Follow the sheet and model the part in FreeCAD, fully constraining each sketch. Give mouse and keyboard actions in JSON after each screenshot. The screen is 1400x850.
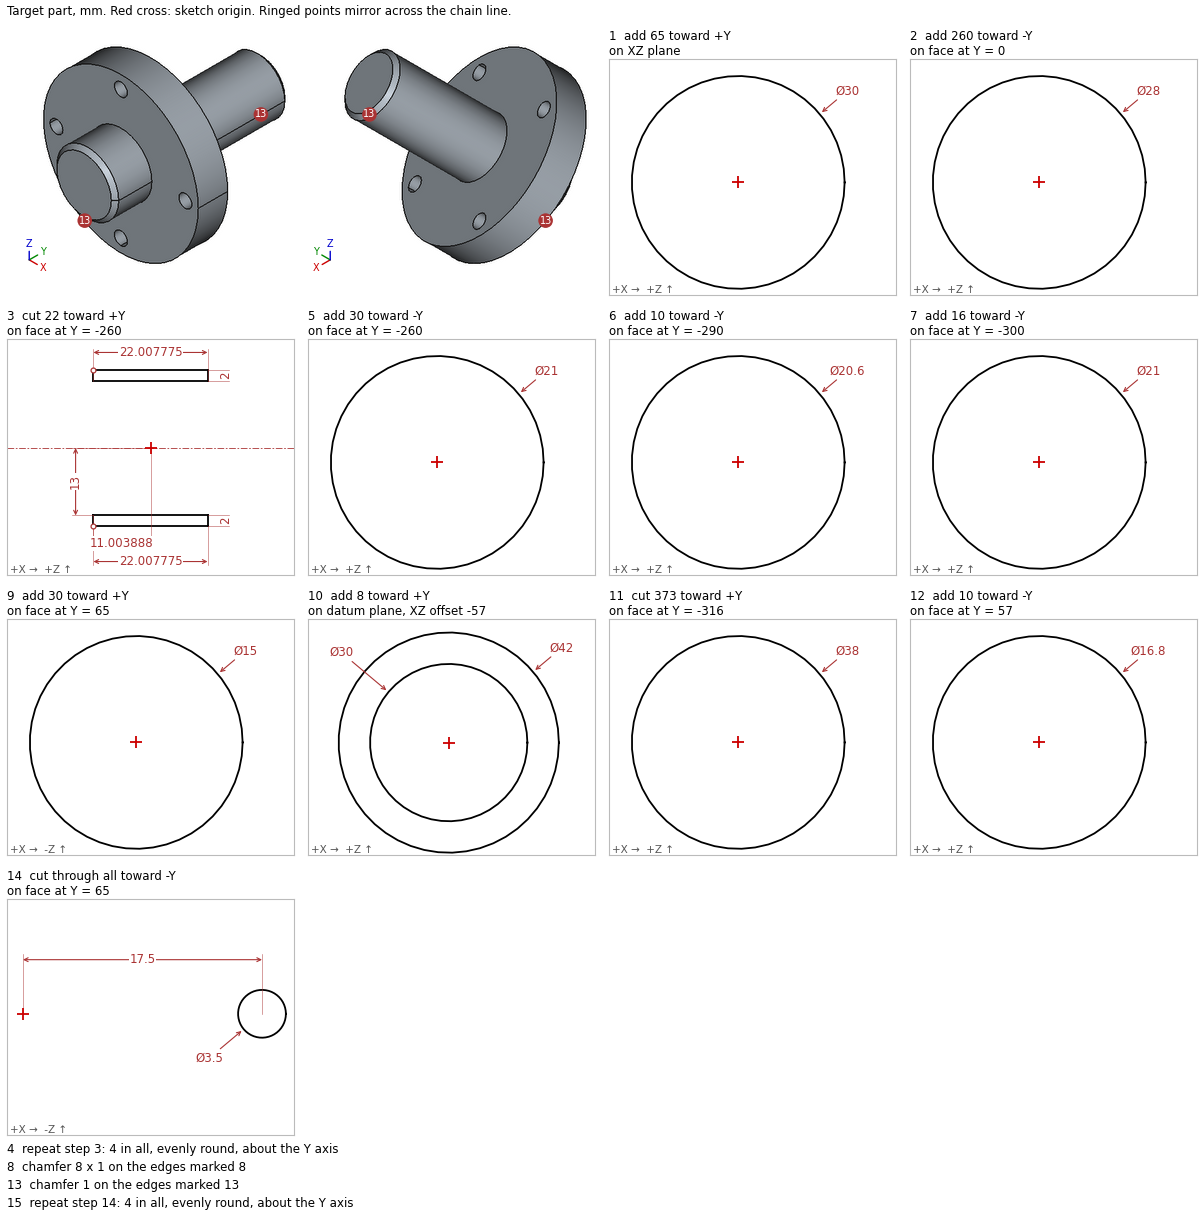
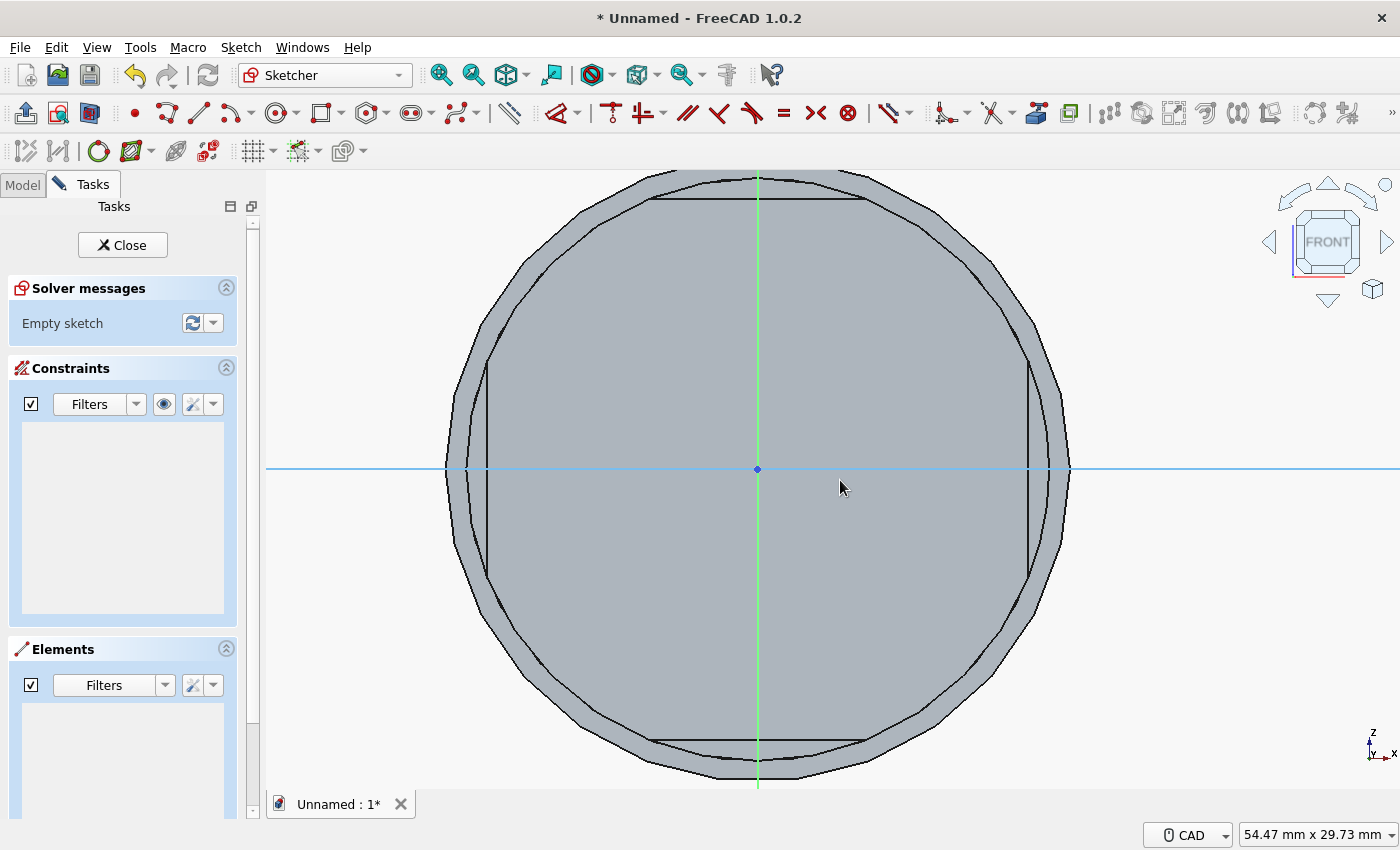
{"action": "left_click", "coordinate": [276, 114]}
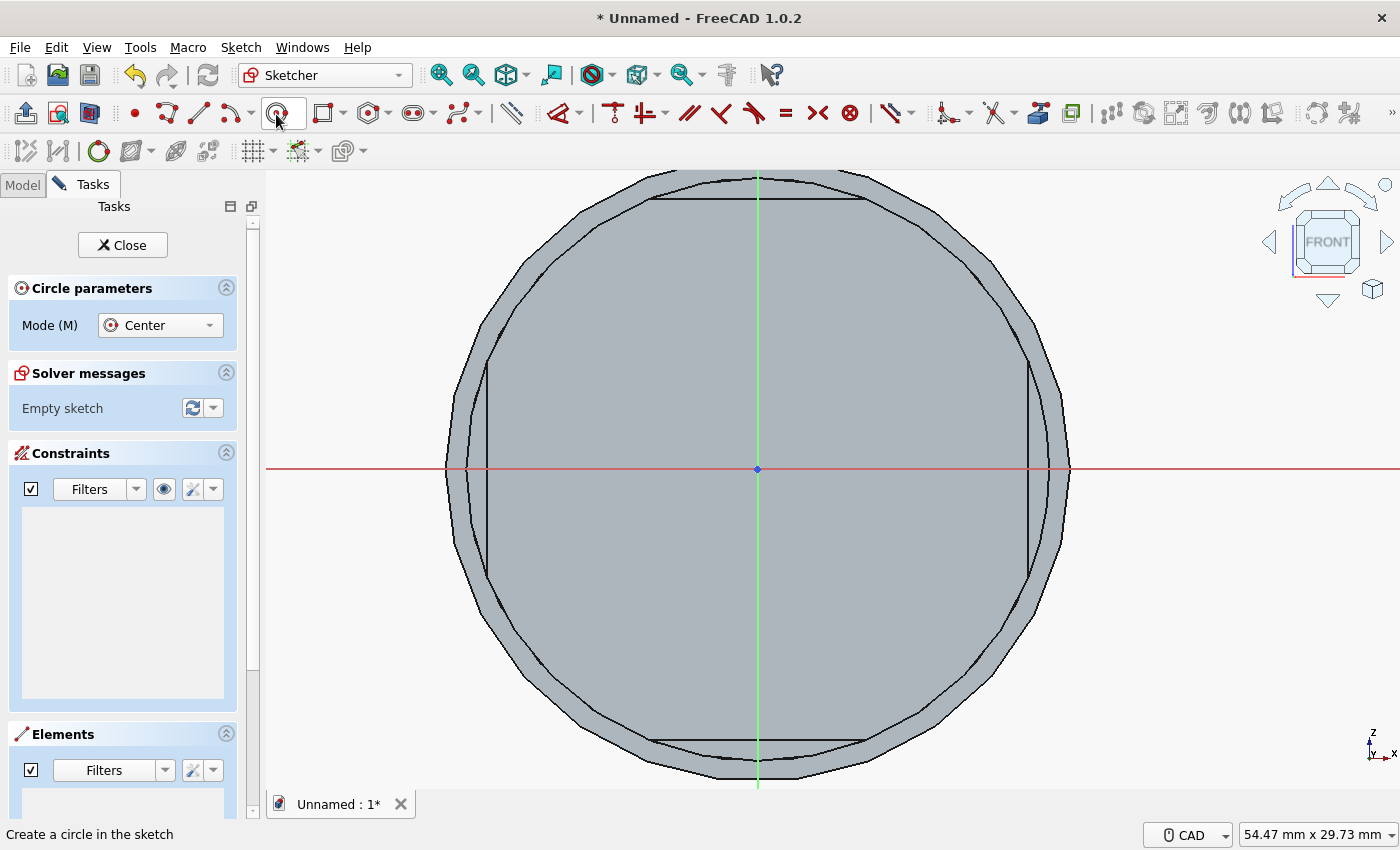
{"action": "left_click", "coordinate": [758, 469]}
{"action": "mouse_move", "coordinate": [912, 315]}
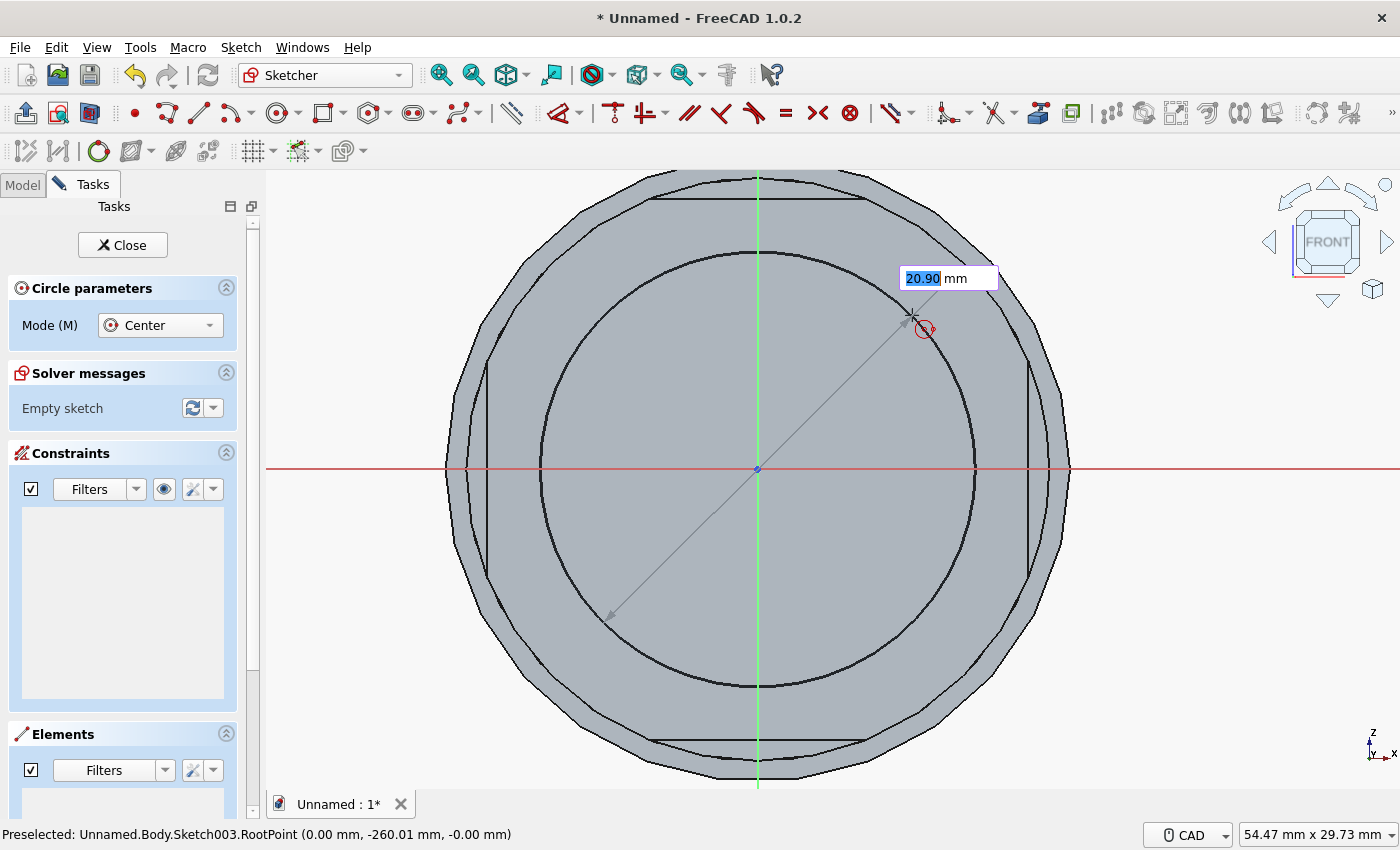
{"action": "type", "text": "21"}
{"action": "key", "text": "Return"}
{"action": "key", "text": "Escape"}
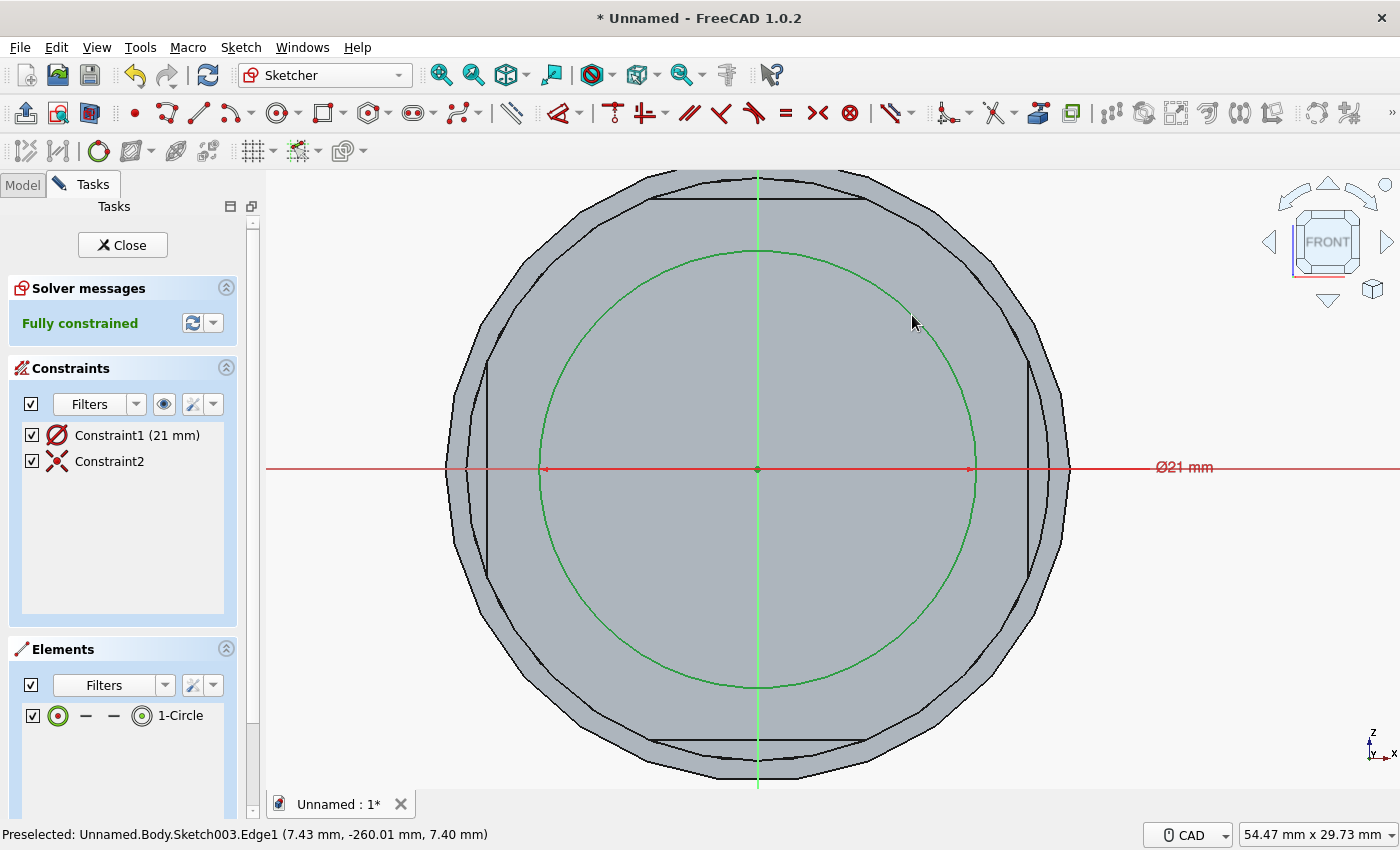
{"action": "left_click", "coordinate": [123, 245]}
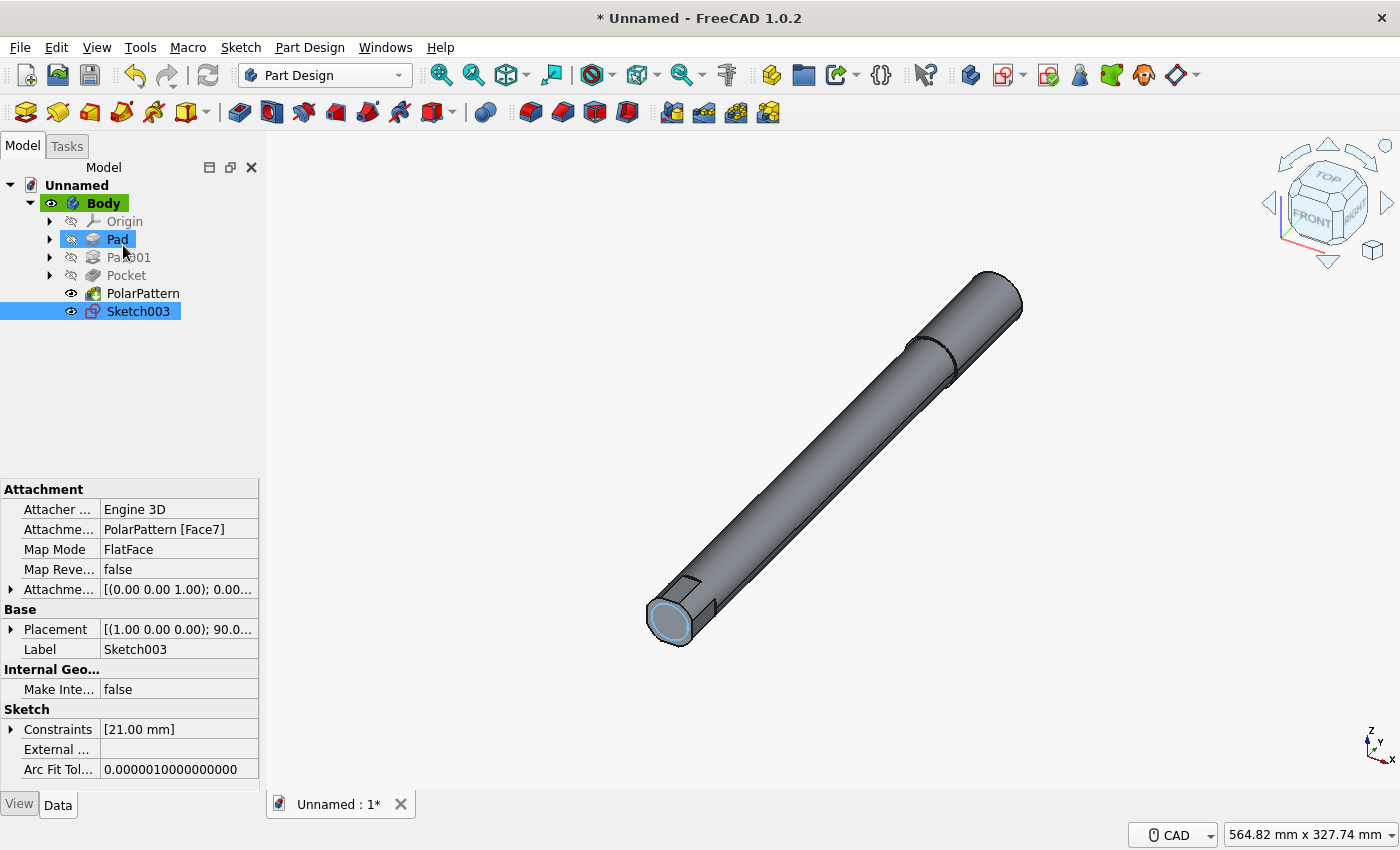
{"action": "left_click", "coordinate": [26, 112]}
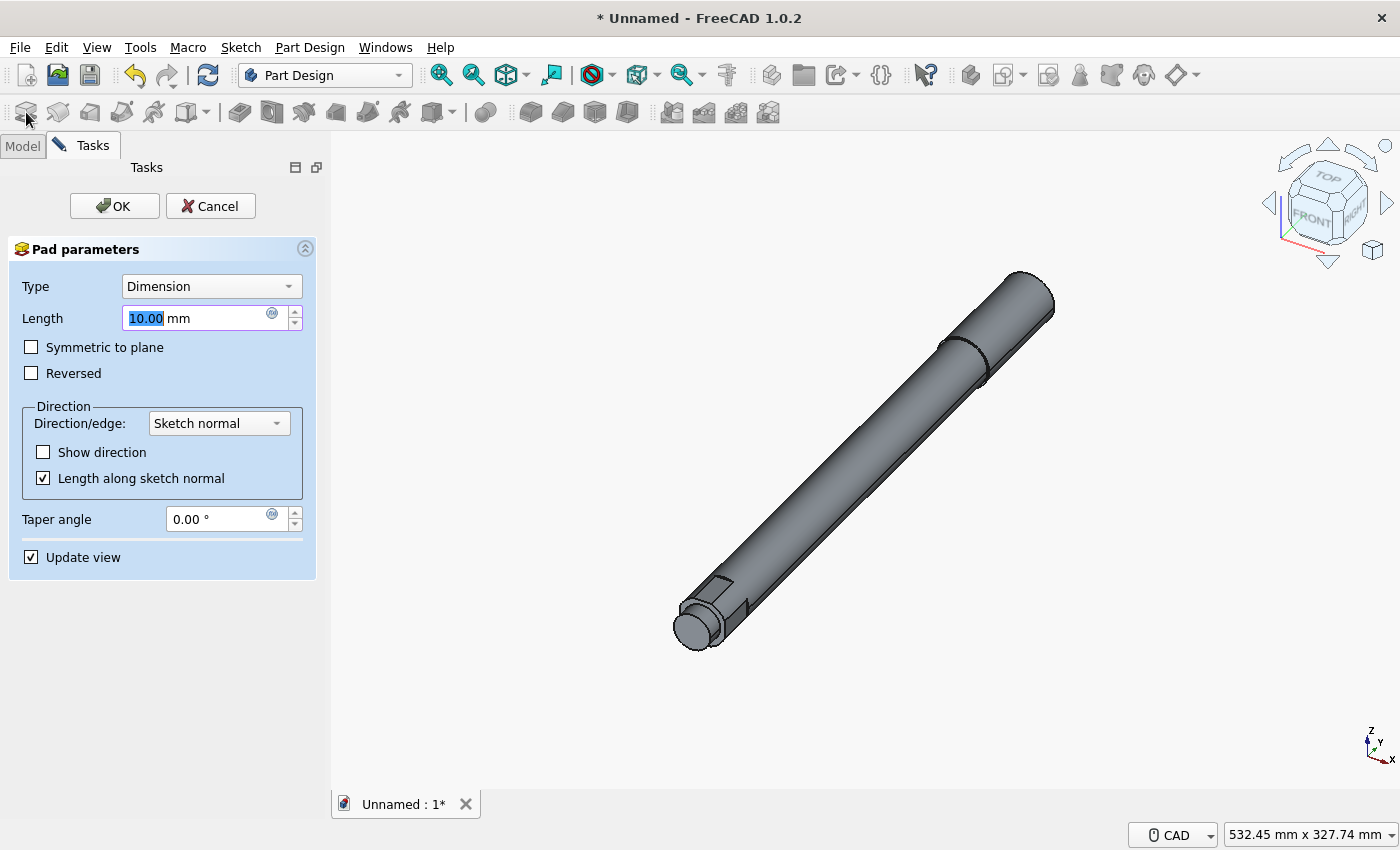
{"action": "type", "text": "30"}
{"action": "key", "text": "Tab"}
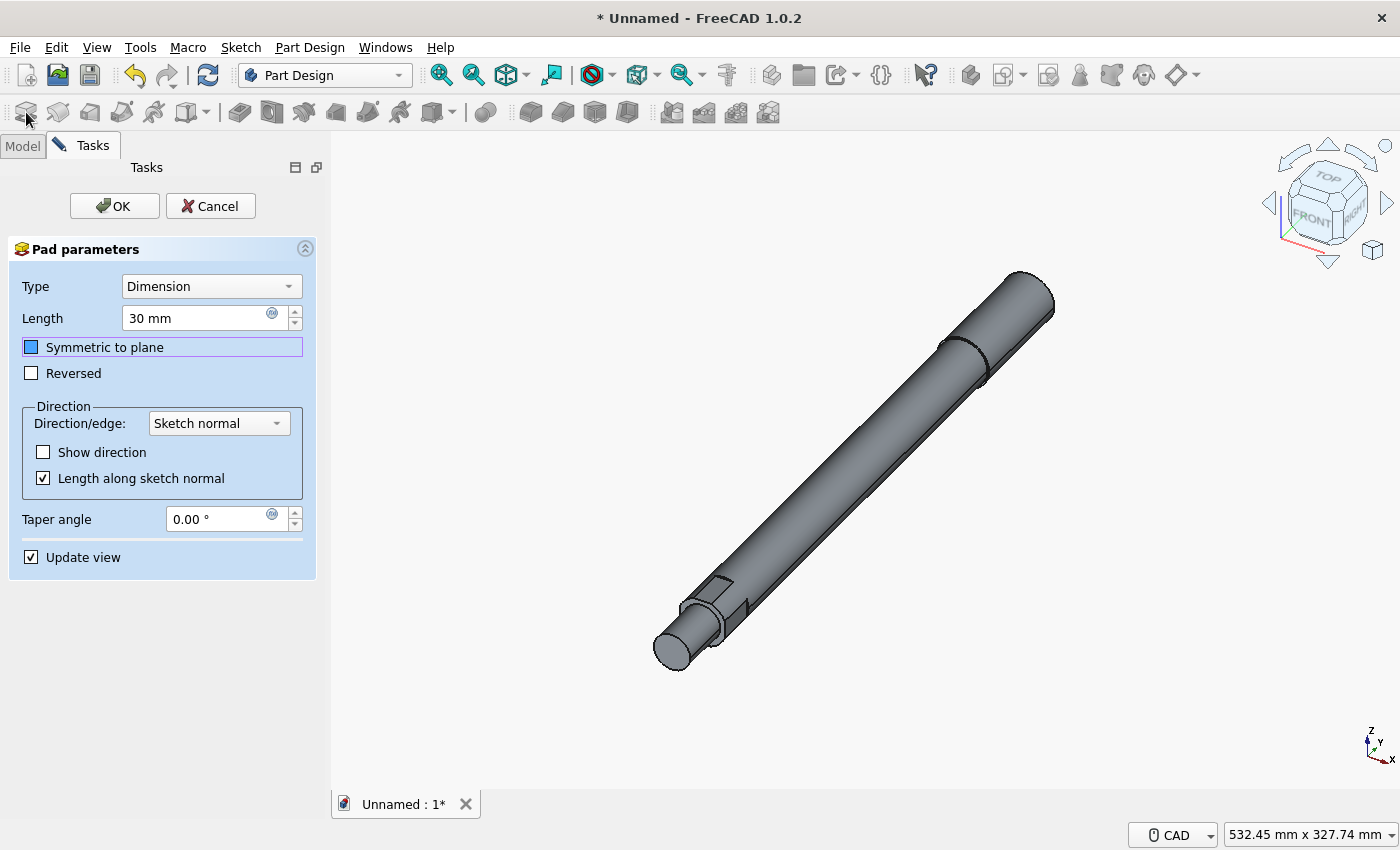
{"action": "left_click", "coordinate": [115, 206]}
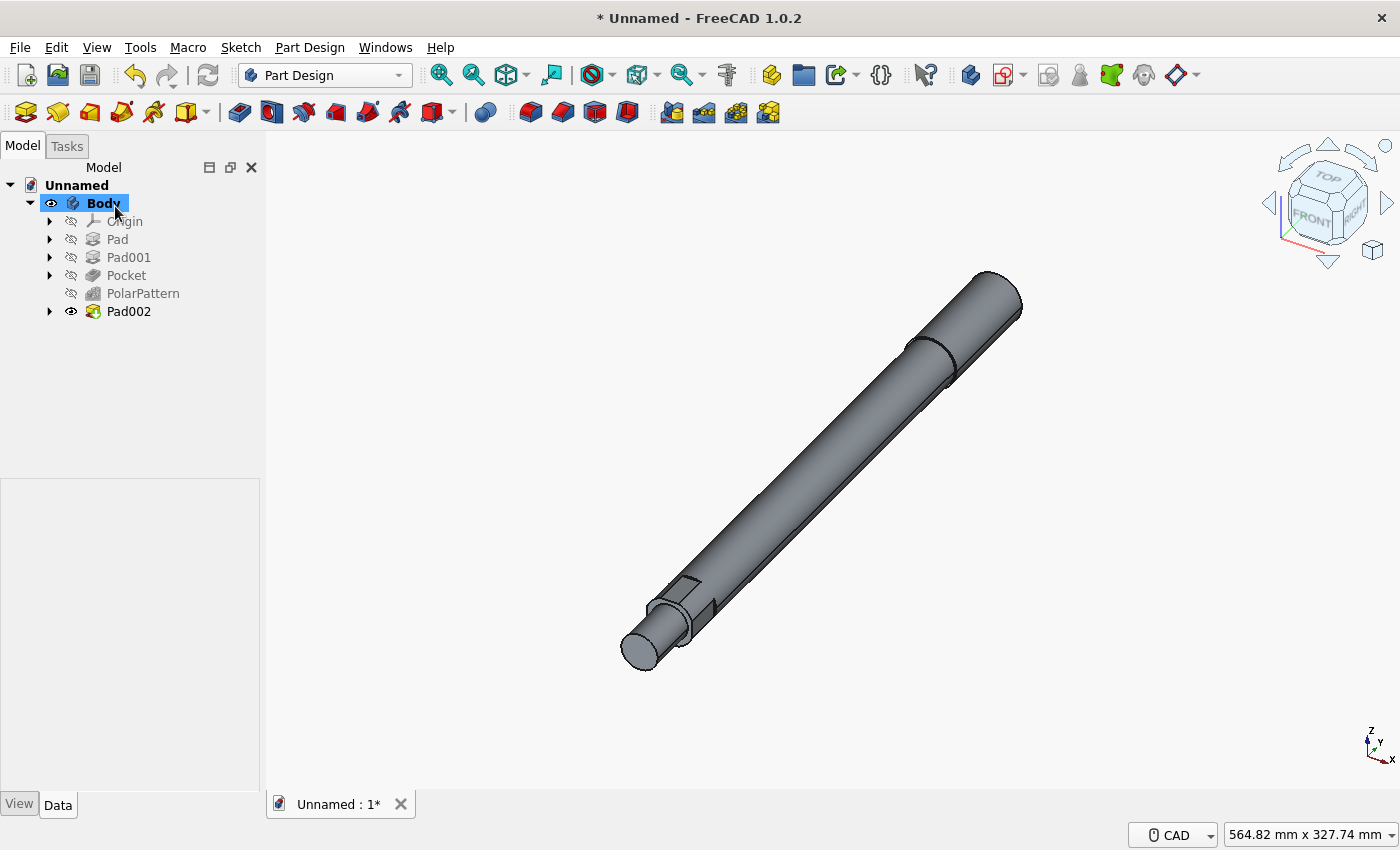
{"action": "left_click", "coordinate": [639, 651]}